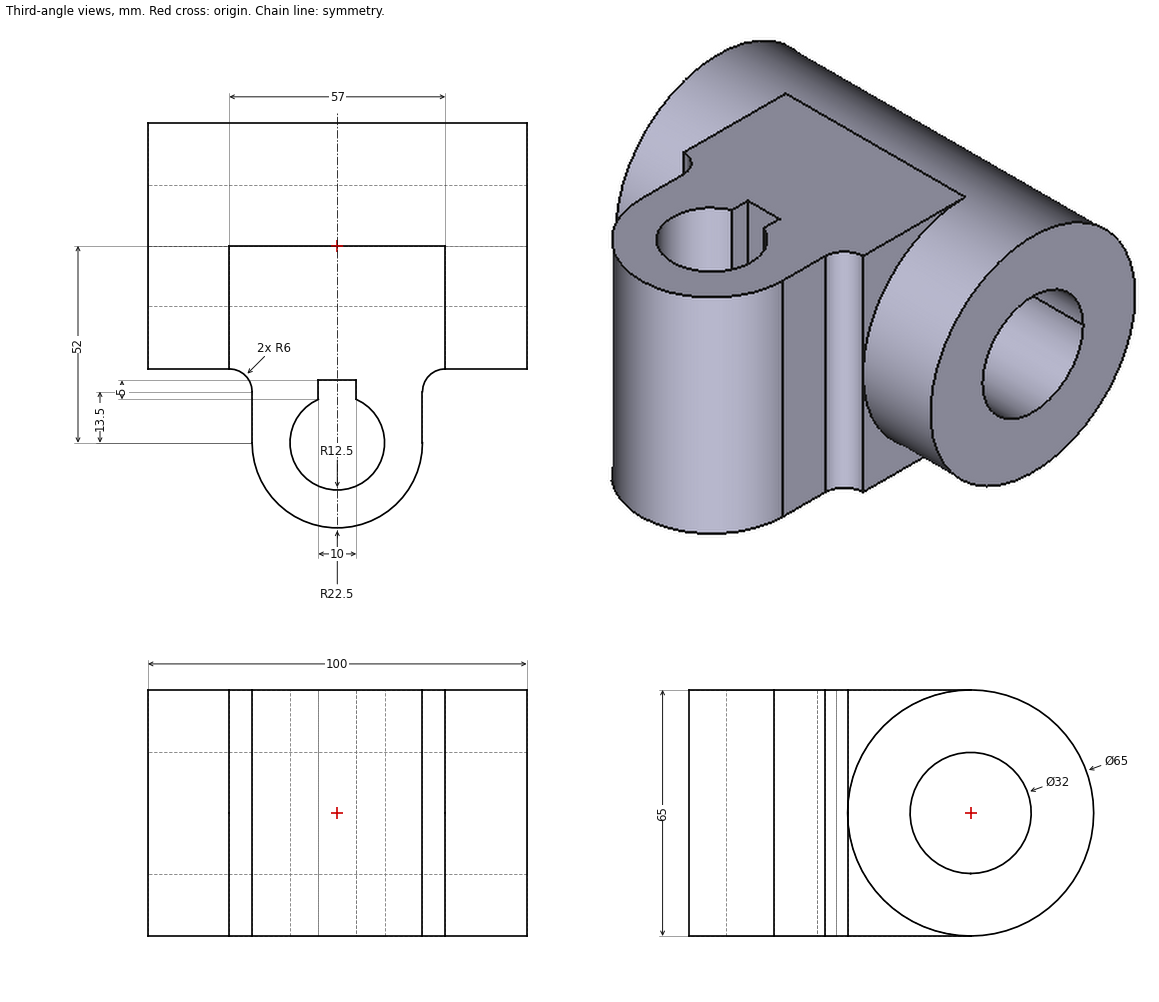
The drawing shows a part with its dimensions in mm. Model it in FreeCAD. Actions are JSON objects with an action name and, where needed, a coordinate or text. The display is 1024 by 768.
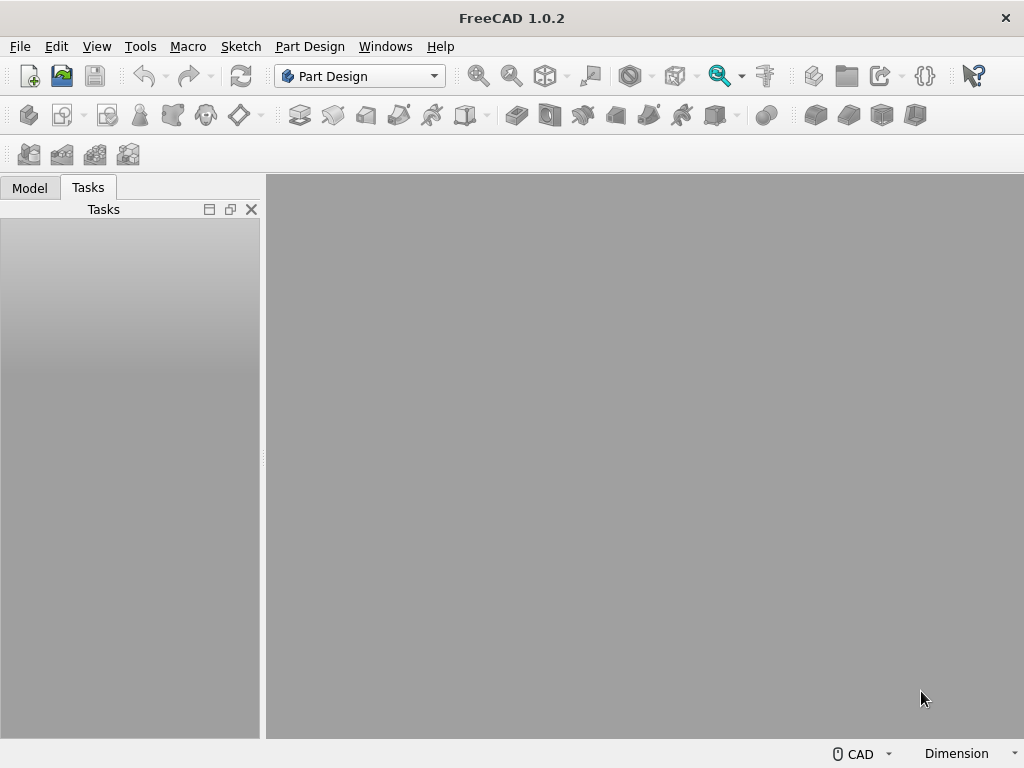
{"action": "left_click", "coordinate": [29, 76]}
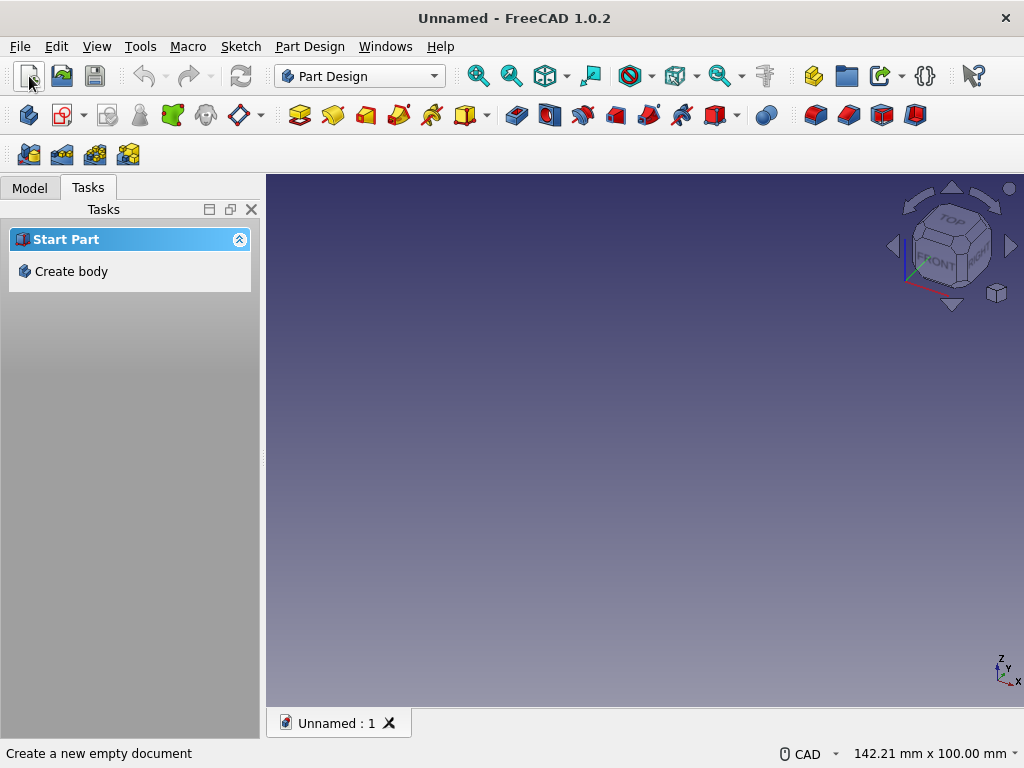
{"action": "left_click", "coordinate": [62, 116]}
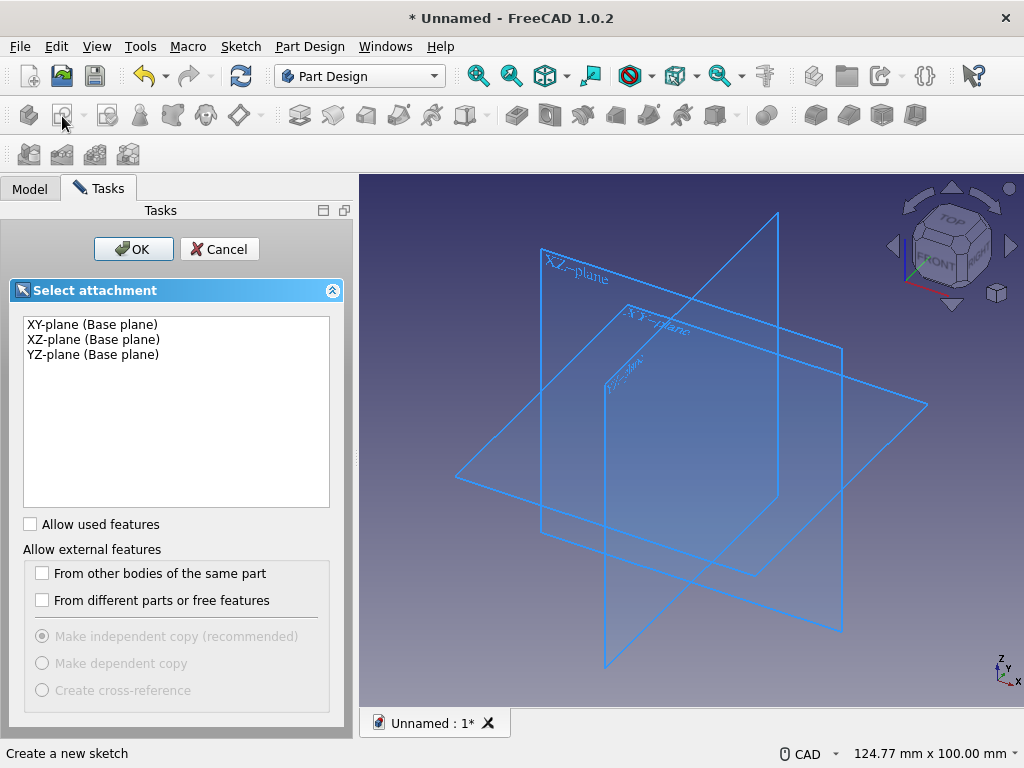
{"action": "left_click", "coordinate": [84, 354]}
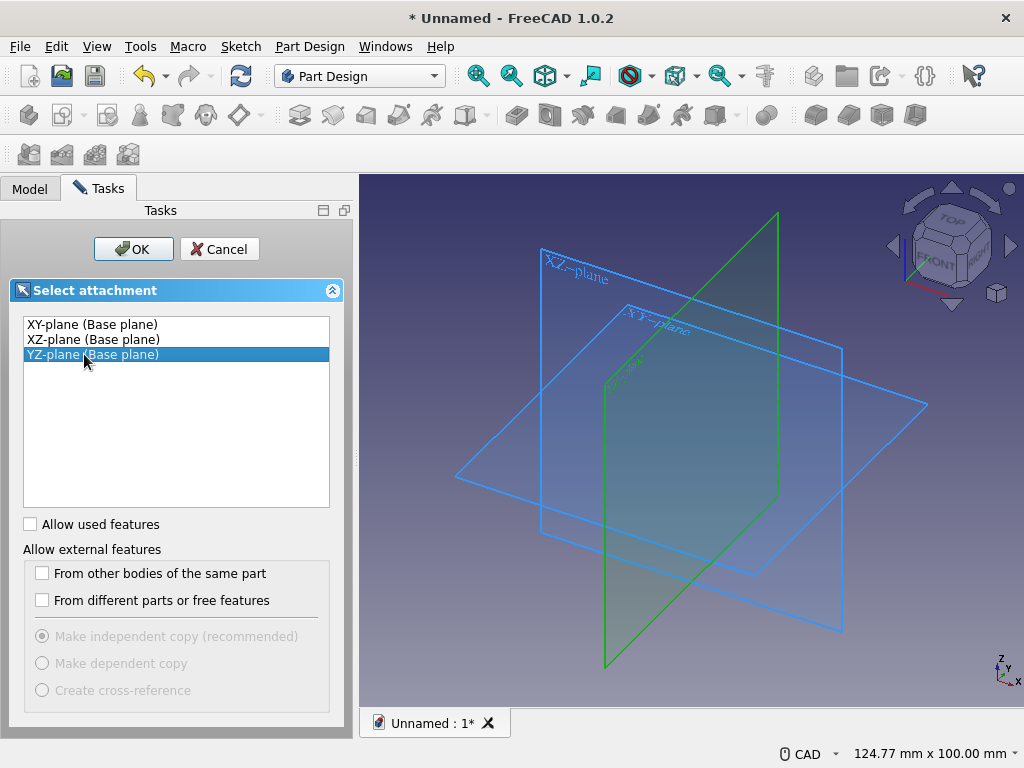
{"action": "left_click", "coordinate": [134, 249]}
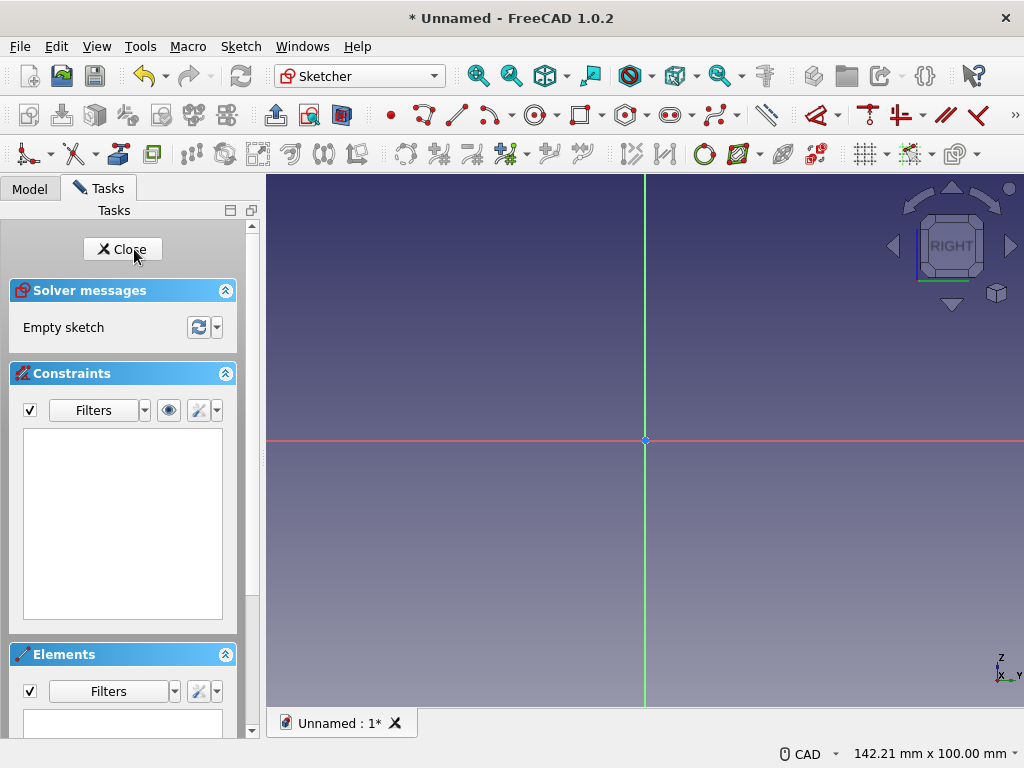
{"action": "key", "text": "g c"}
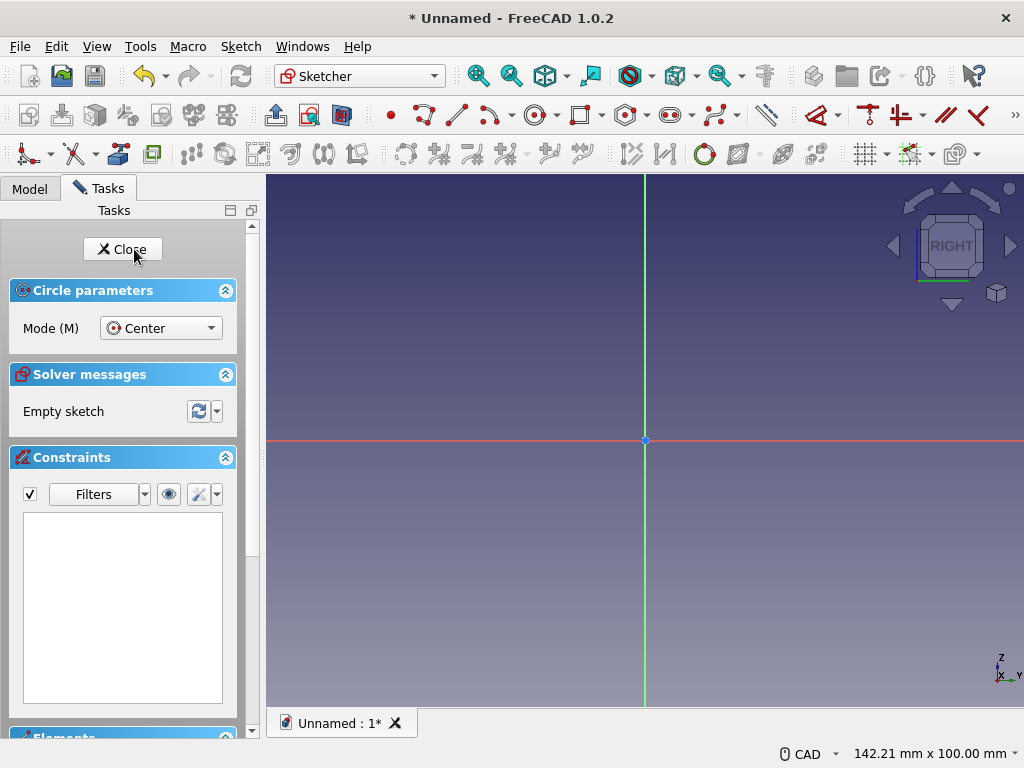
{"action": "left_click", "coordinate": [645, 440]}
{"action": "mouse_move", "coordinate": [767, 318]}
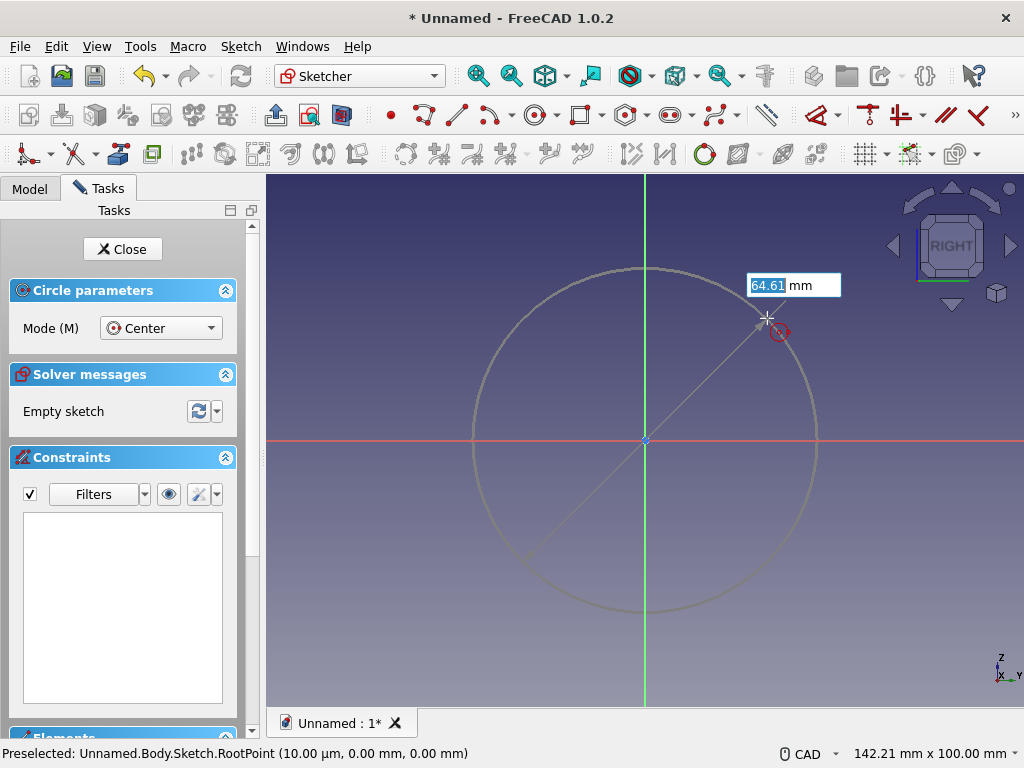
{"action": "type", "text": "65"}
{"action": "key", "text": "Return"}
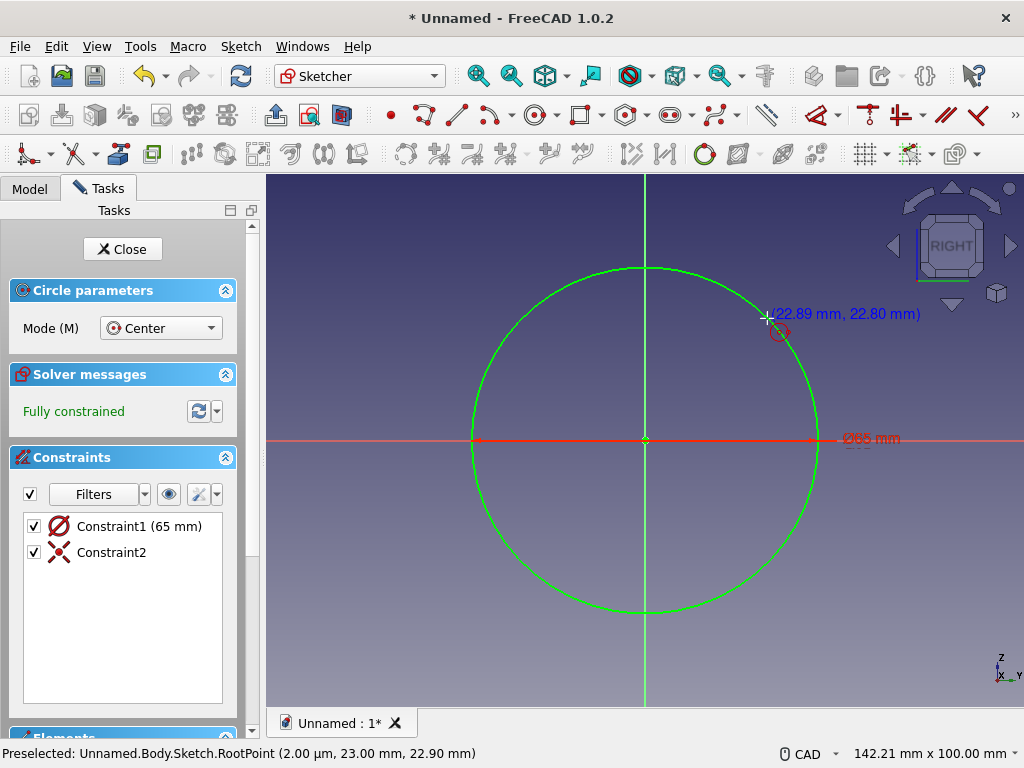
{"action": "left_click", "coordinate": [645, 440]}
{"action": "mouse_move", "coordinate": [705, 380]}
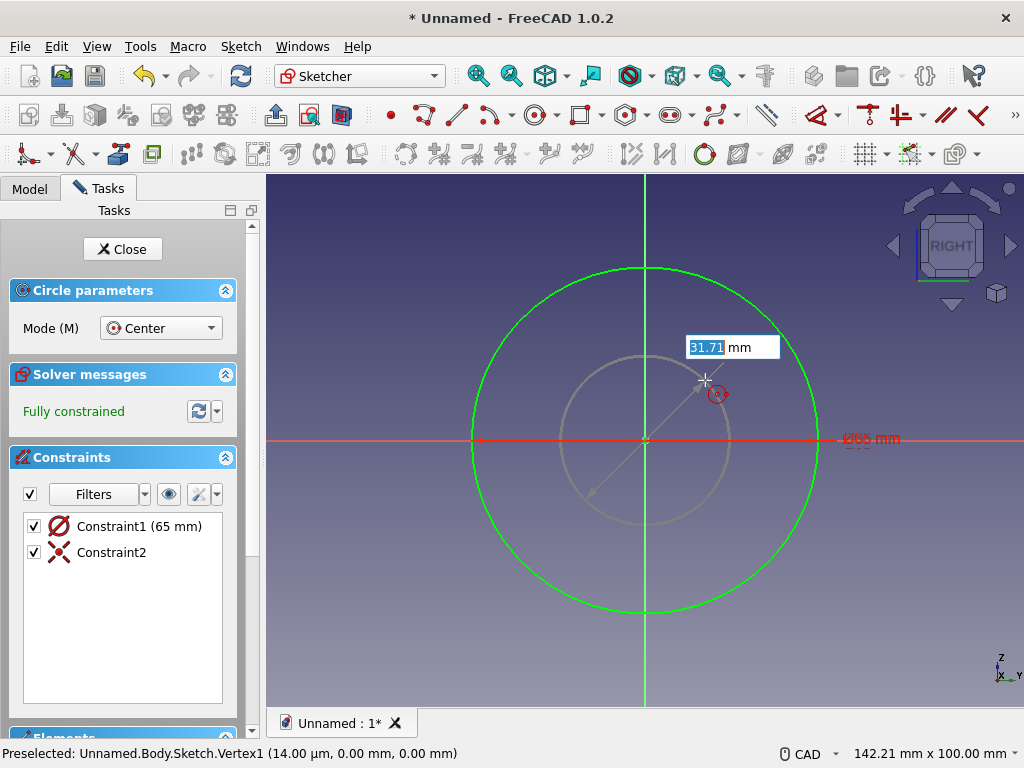
{"action": "type", "text": "32"}
{"action": "key", "text": "Return"}
{"action": "key", "text": "Escape"}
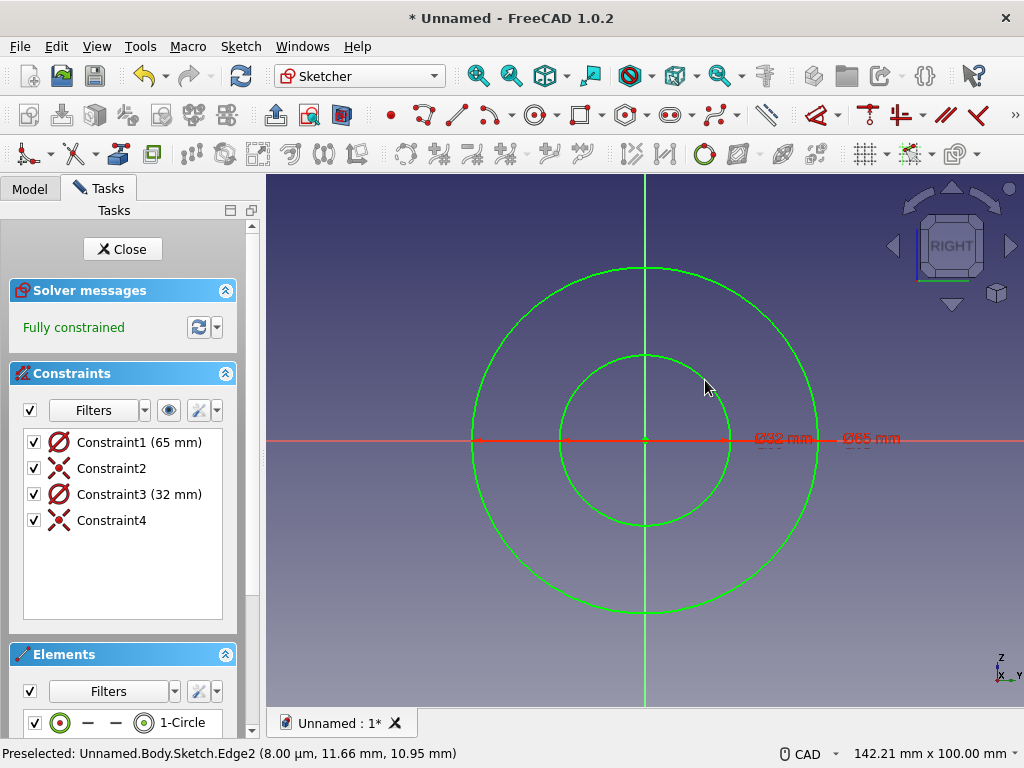
{"action": "left_click", "coordinate": [123, 249]}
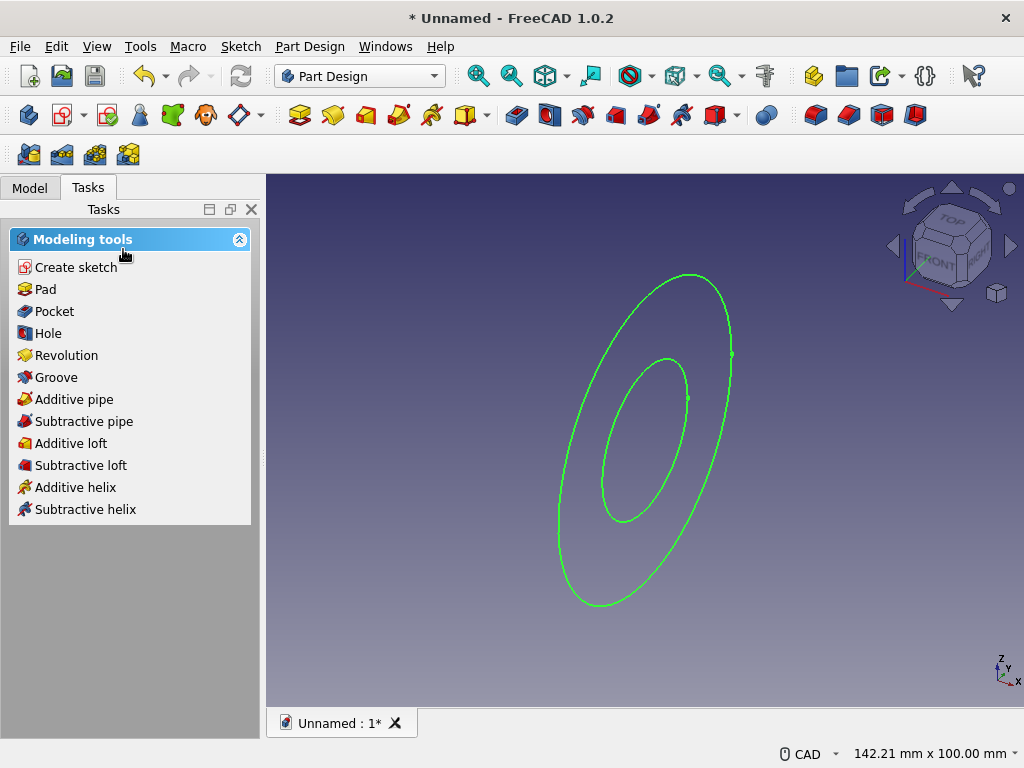
{"action": "left_click", "coordinate": [300, 116]}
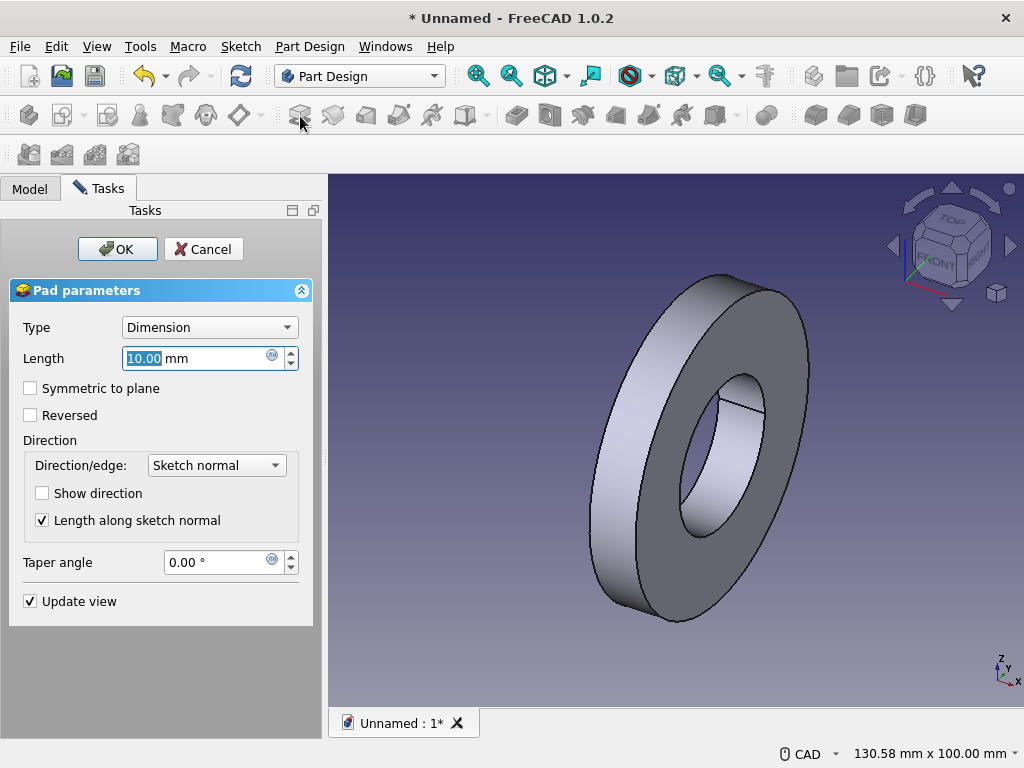
{"action": "type", "text": "100"}
{"action": "key", "text": "Tab"}